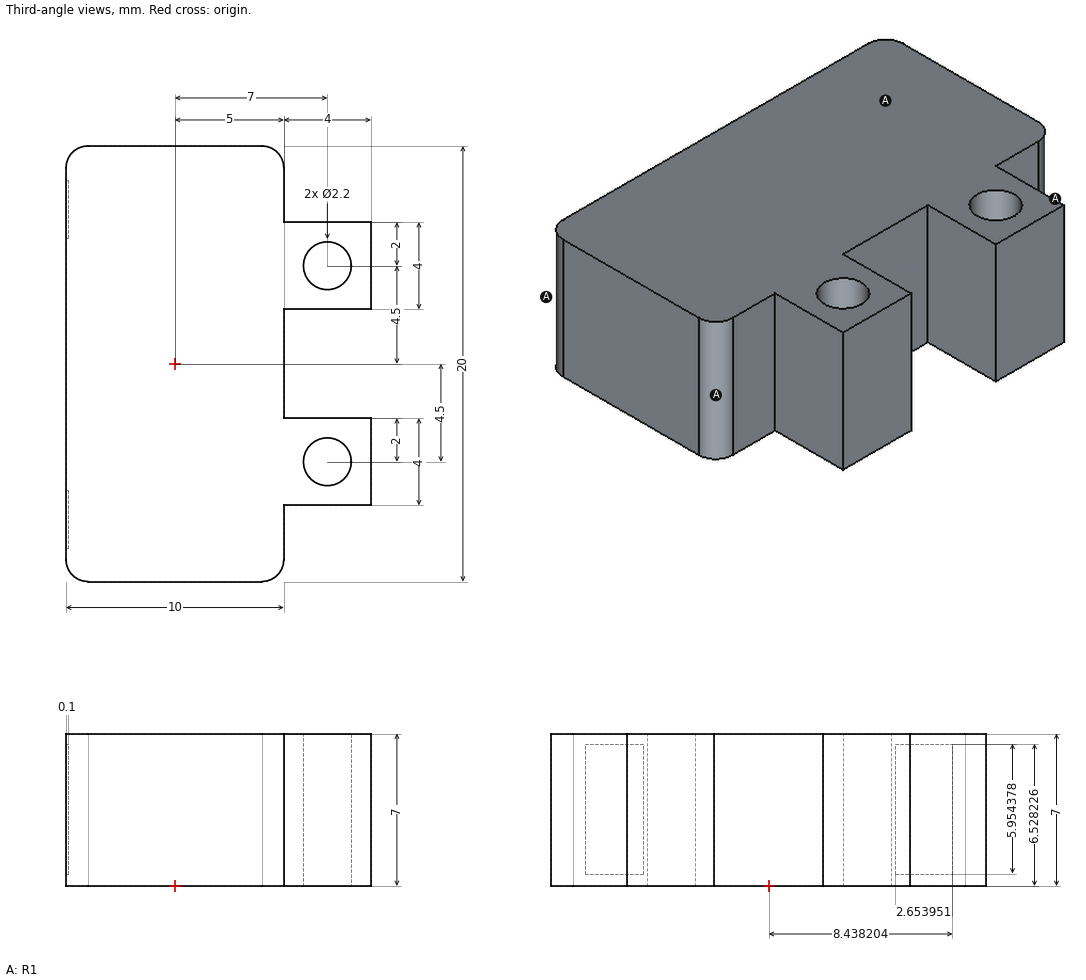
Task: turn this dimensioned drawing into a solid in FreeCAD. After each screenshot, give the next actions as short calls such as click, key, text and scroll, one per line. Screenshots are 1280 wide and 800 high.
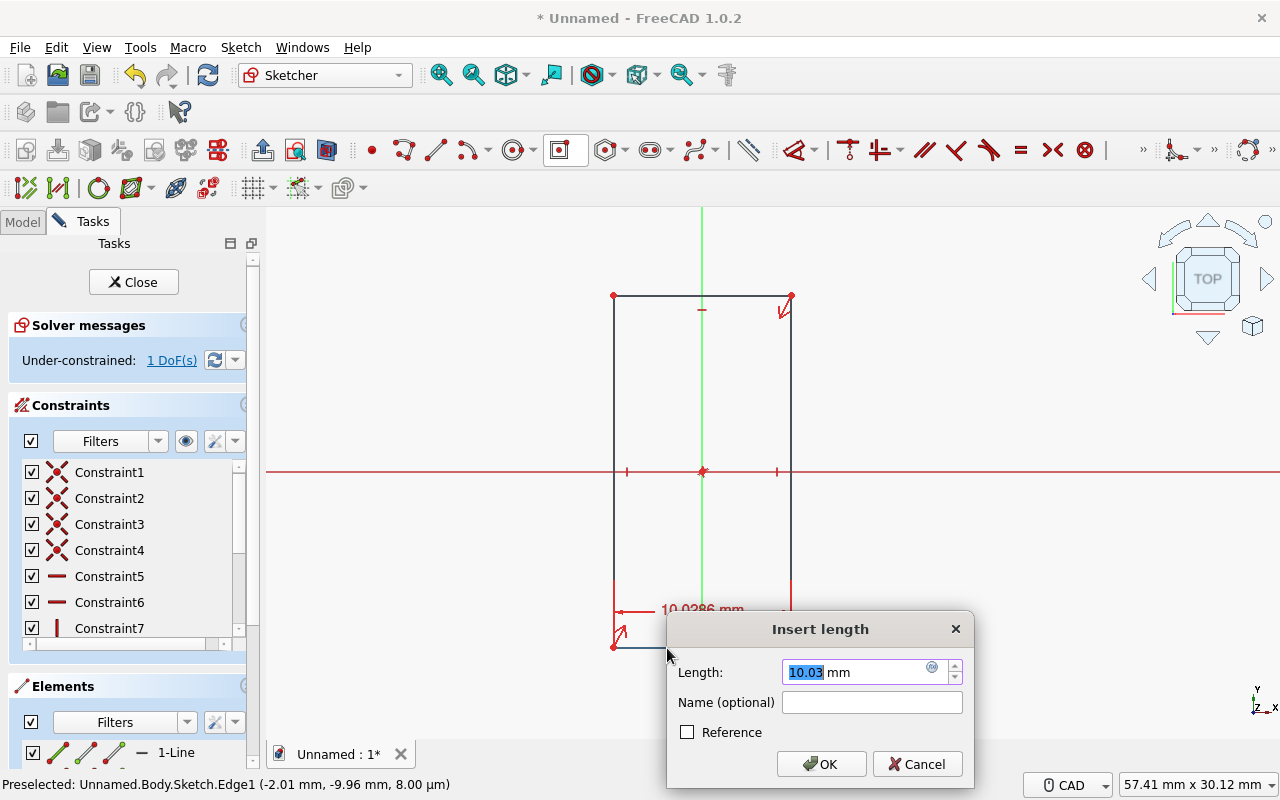
text(10)
key(Return)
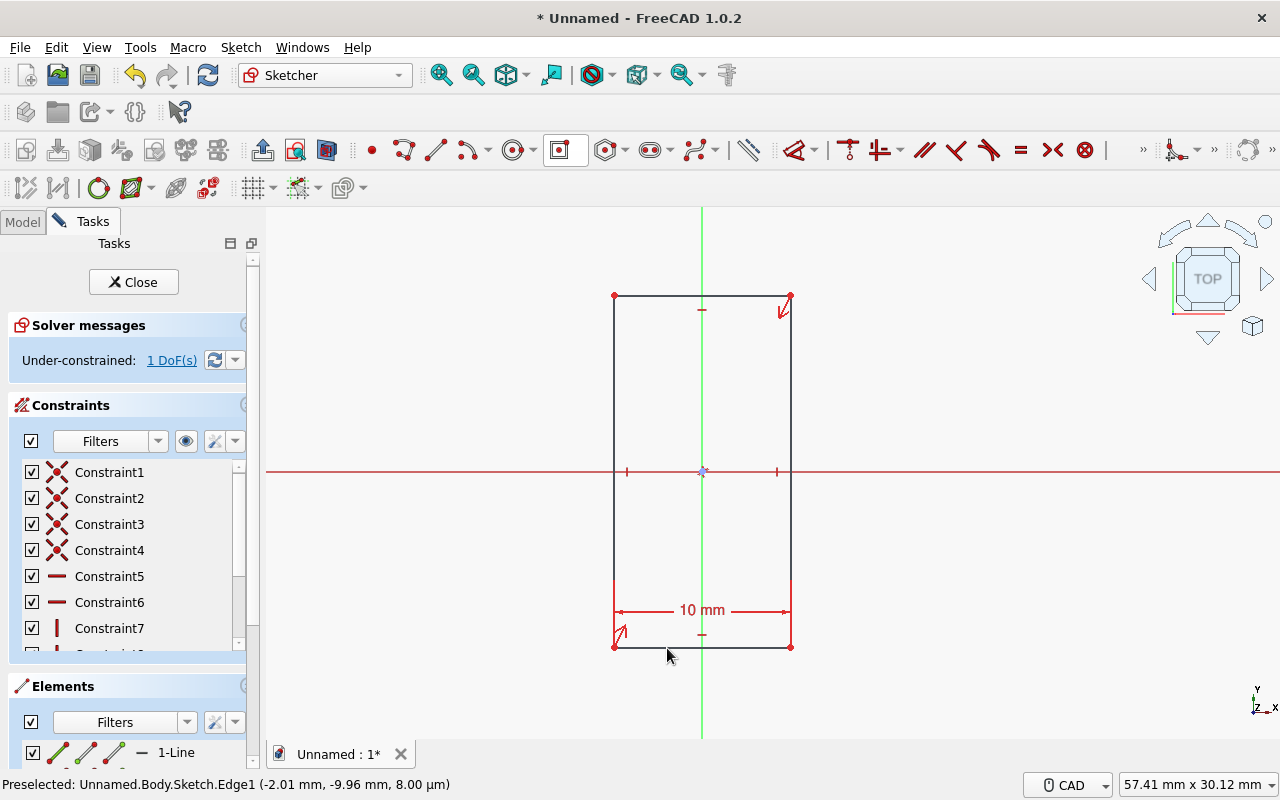
click(791, 542)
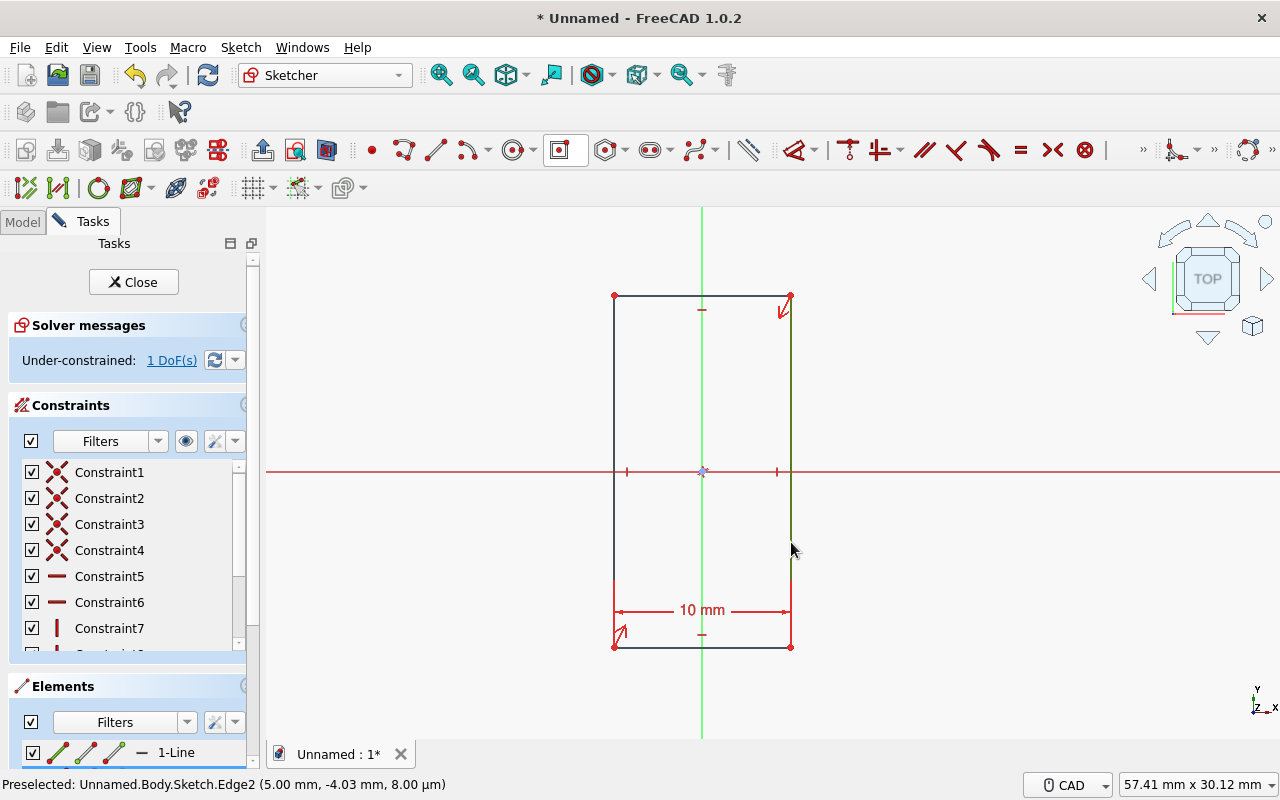
key(i)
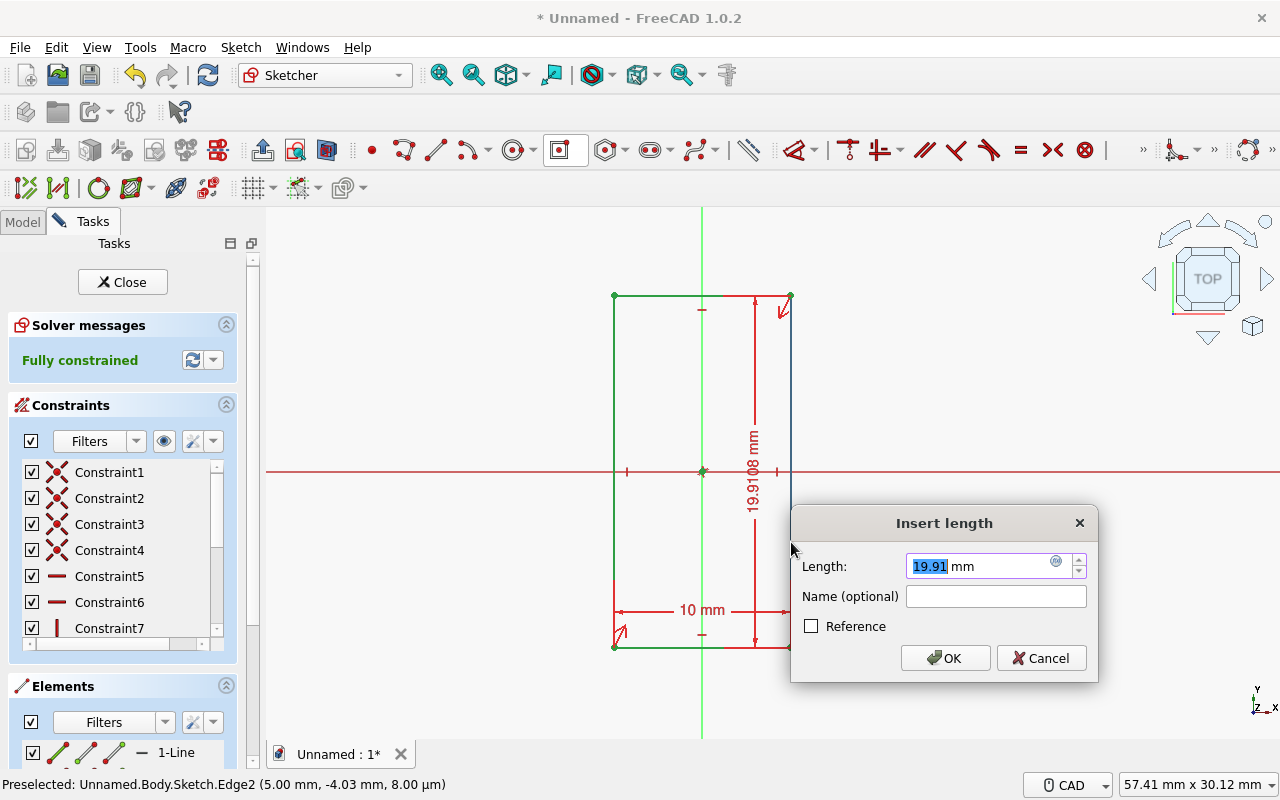
text(20)
key(Return)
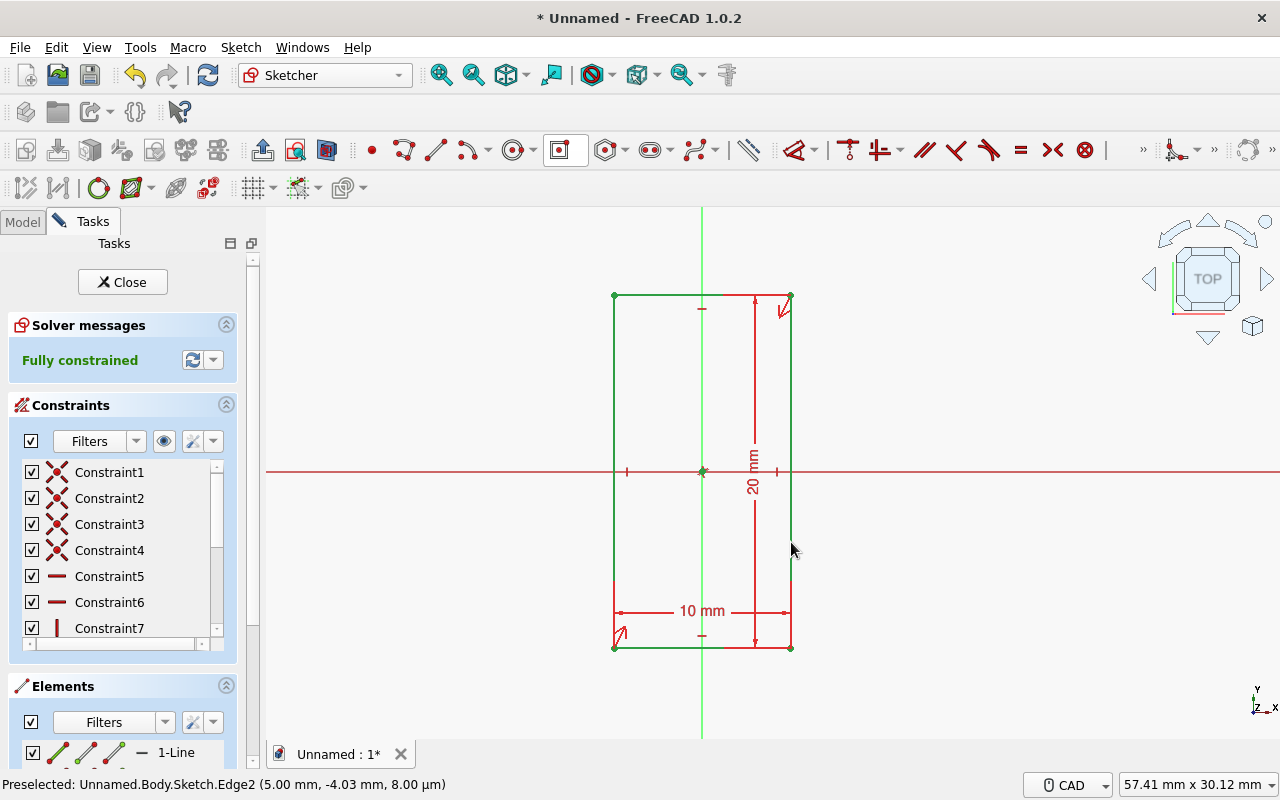
click(123, 282)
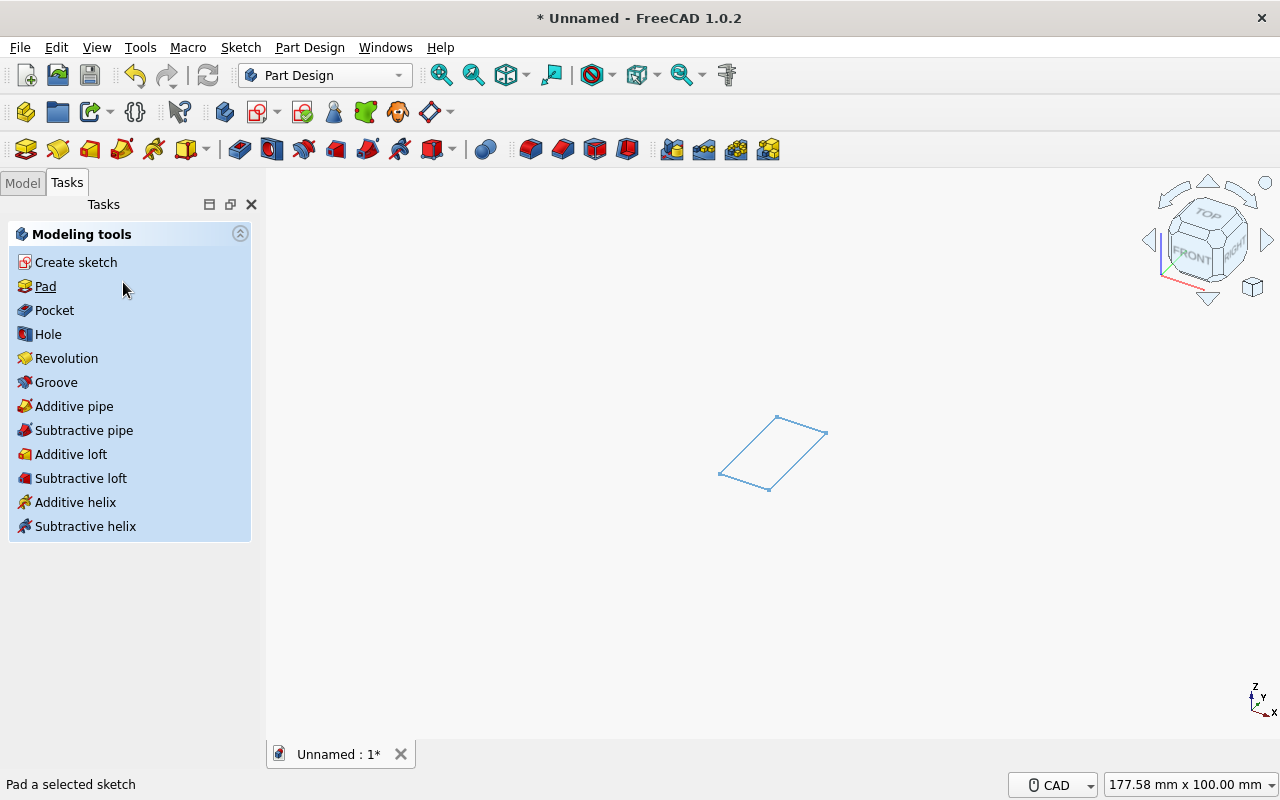
click(26, 150)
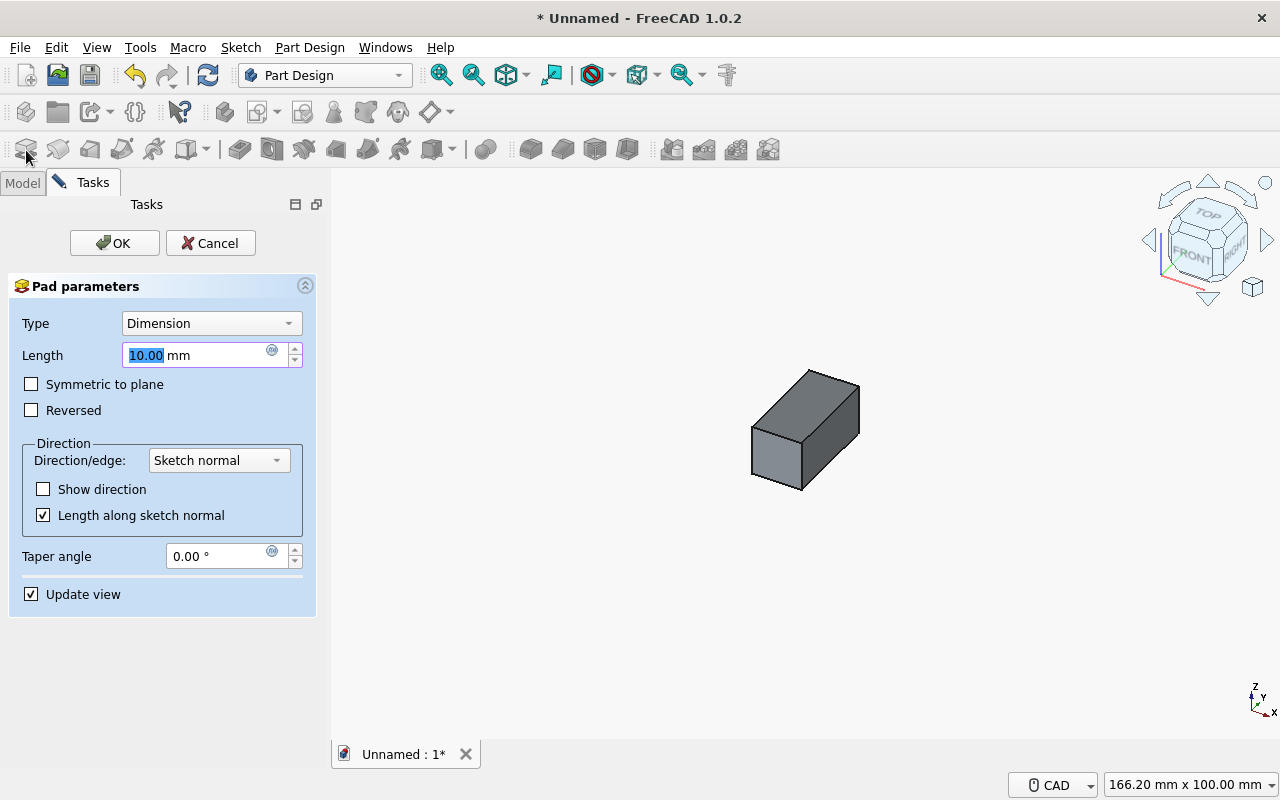
text(7)
key(Tab)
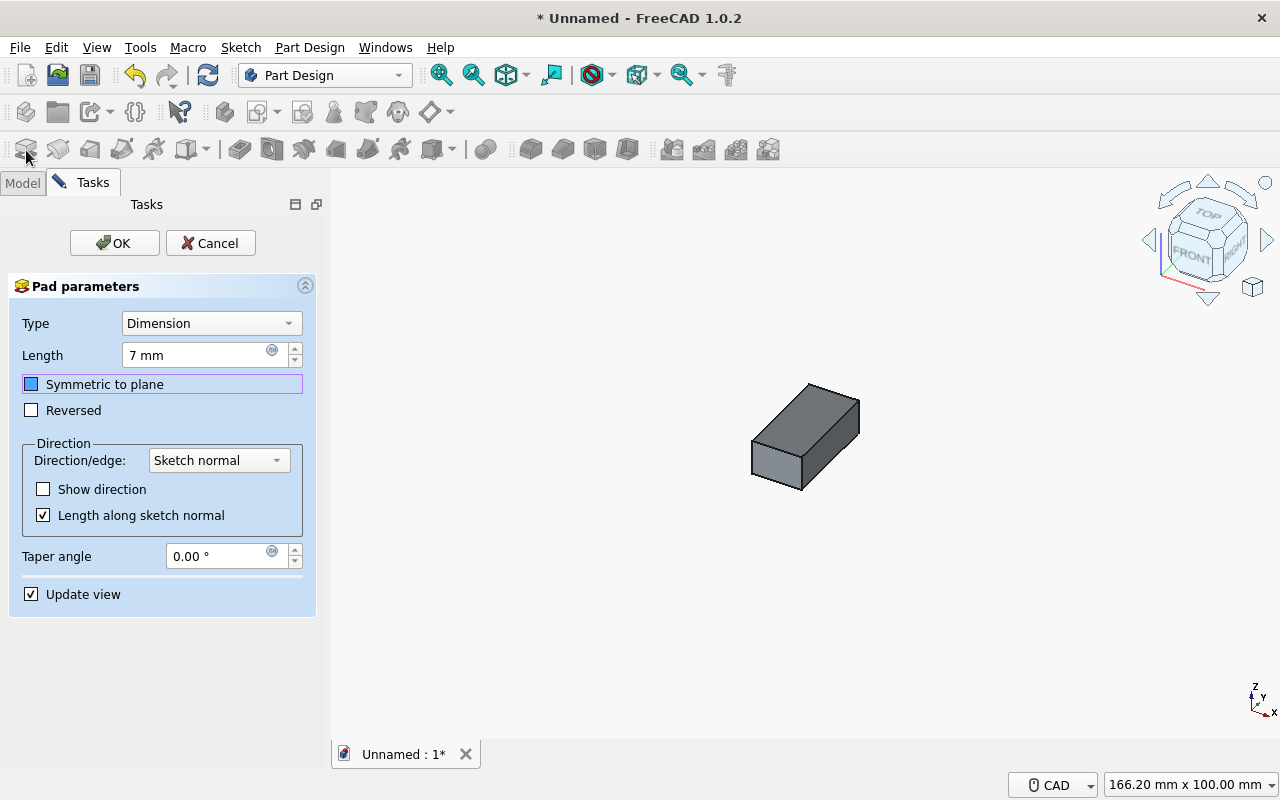
click(115, 243)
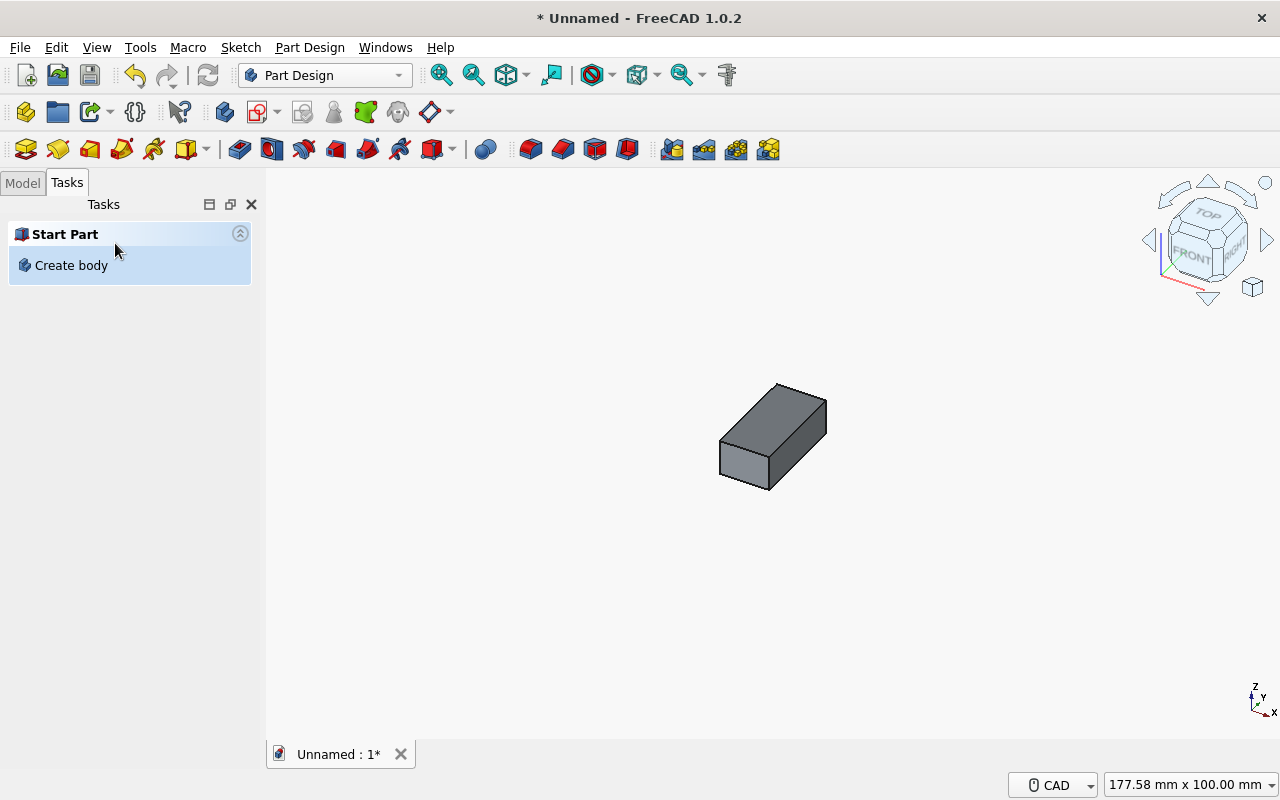
key(v)
key(f)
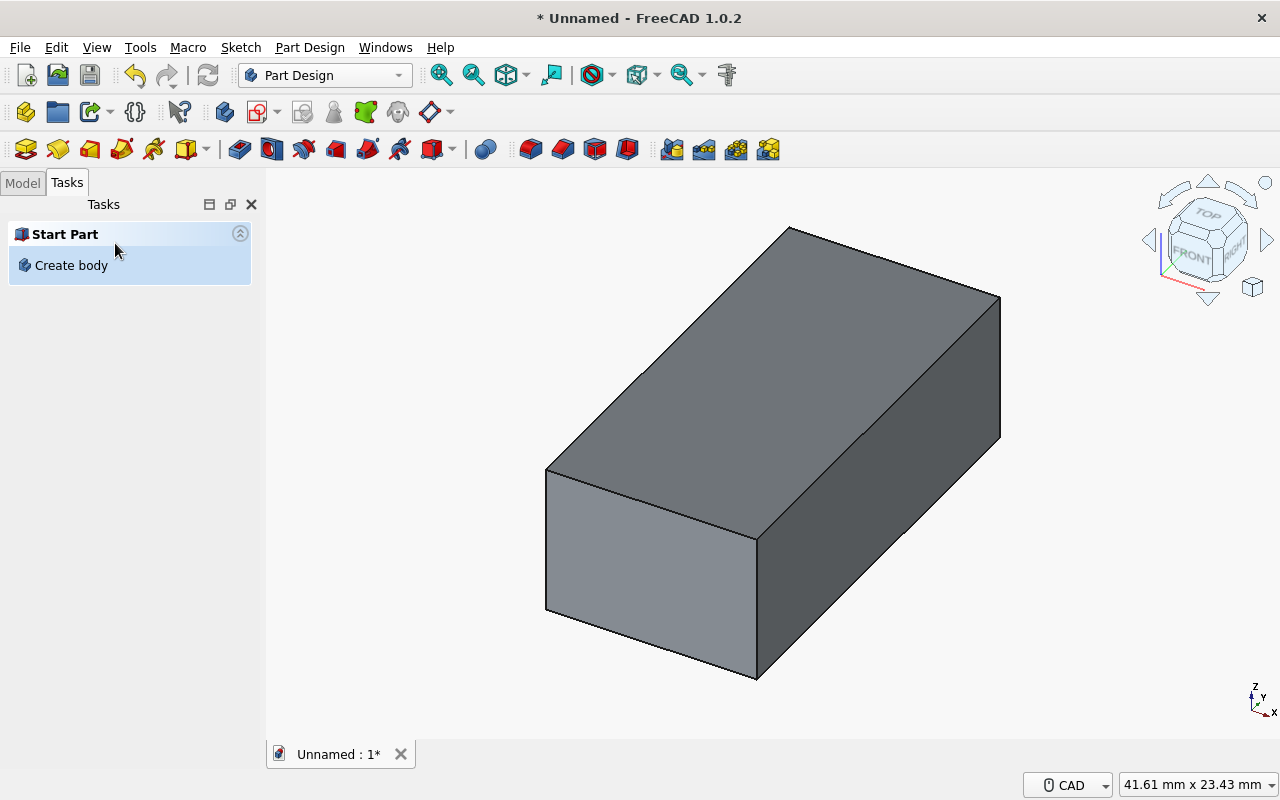
click(808, 348)